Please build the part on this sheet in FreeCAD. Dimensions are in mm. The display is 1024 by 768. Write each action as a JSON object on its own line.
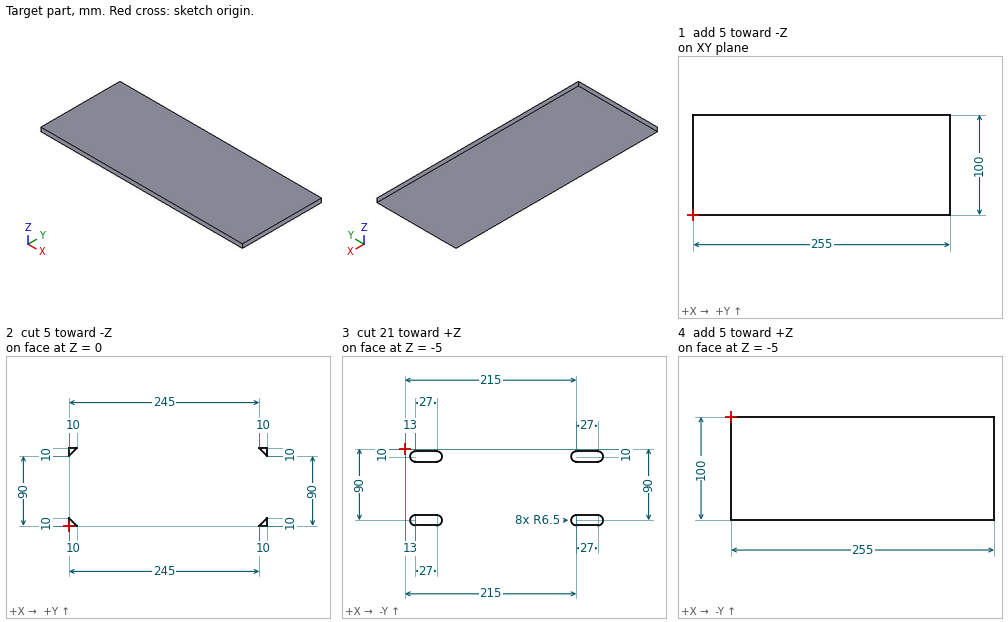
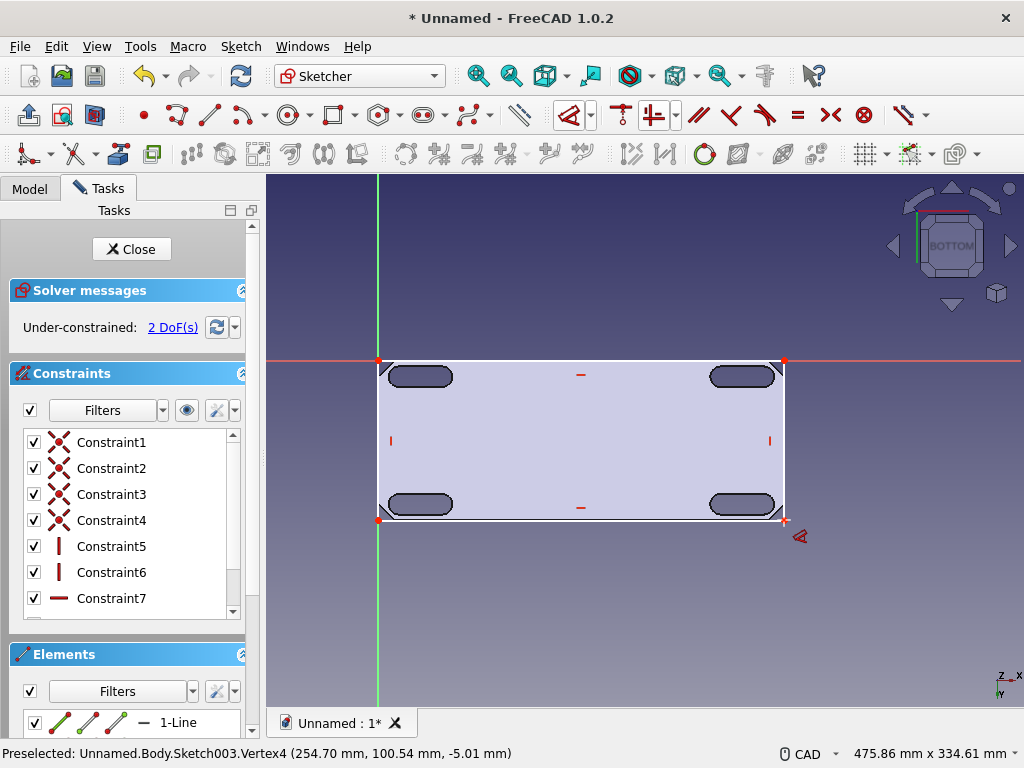
{"action": "left_click", "coordinate": [378, 409]}
{"action": "left_click", "coordinate": [344, 441]}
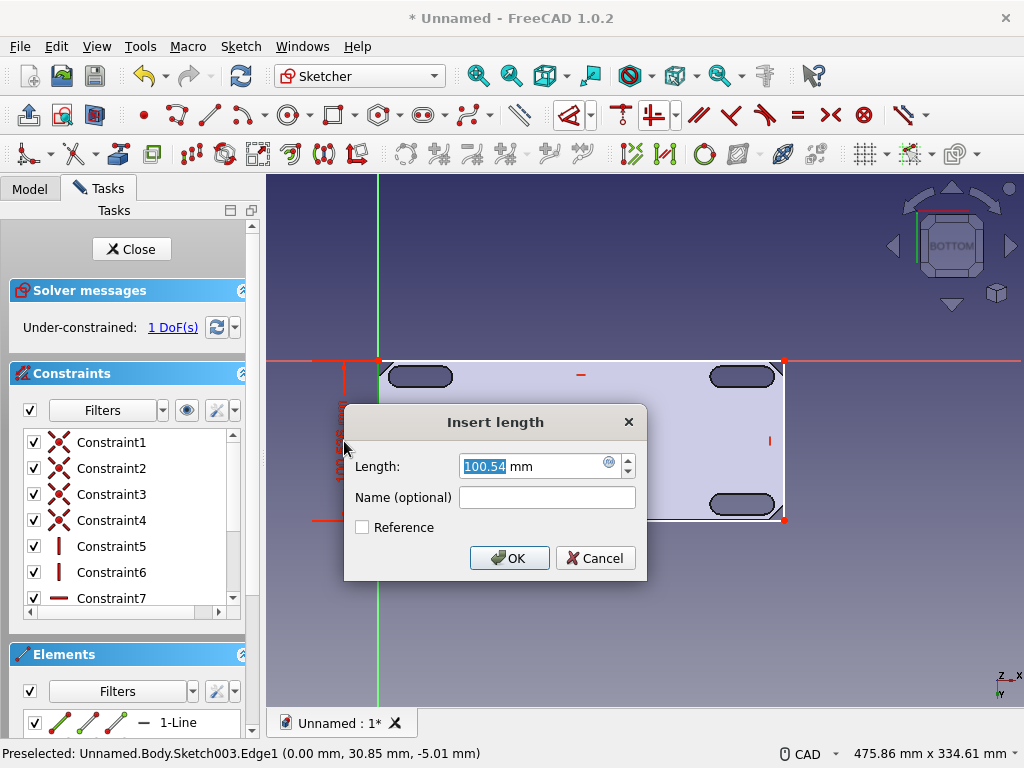
{"action": "type", "text": "100"}
{"action": "key", "text": "Return"}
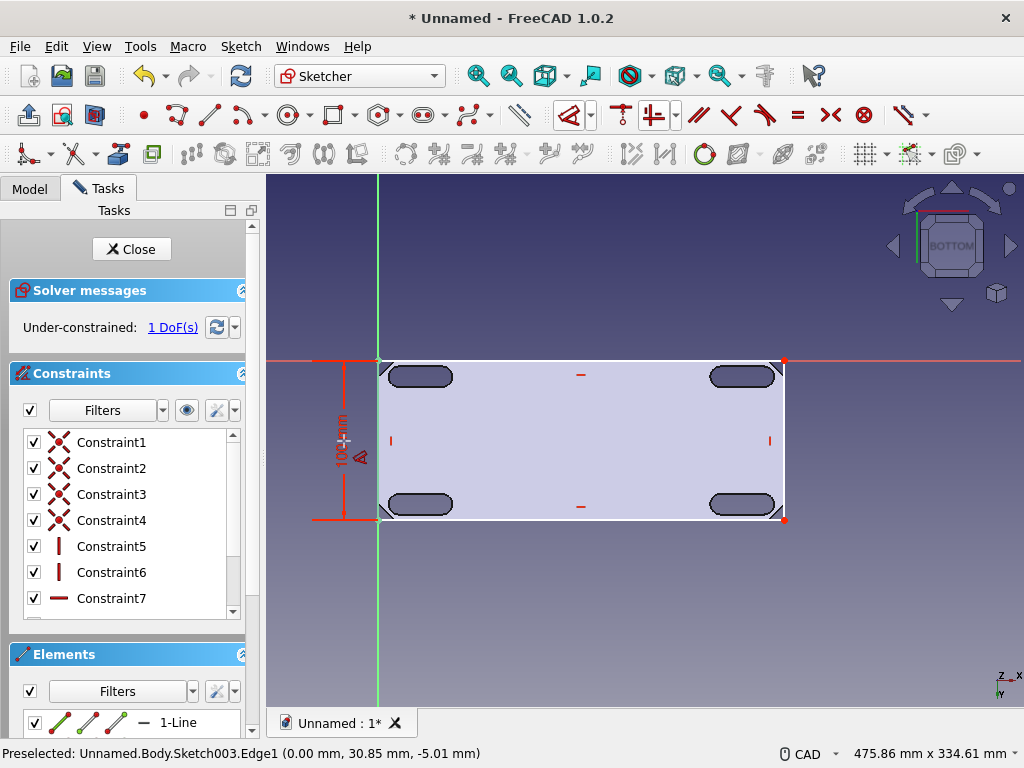
{"action": "left_click", "coordinate": [500, 520]}
{"action": "left_click", "coordinate": [581, 554]}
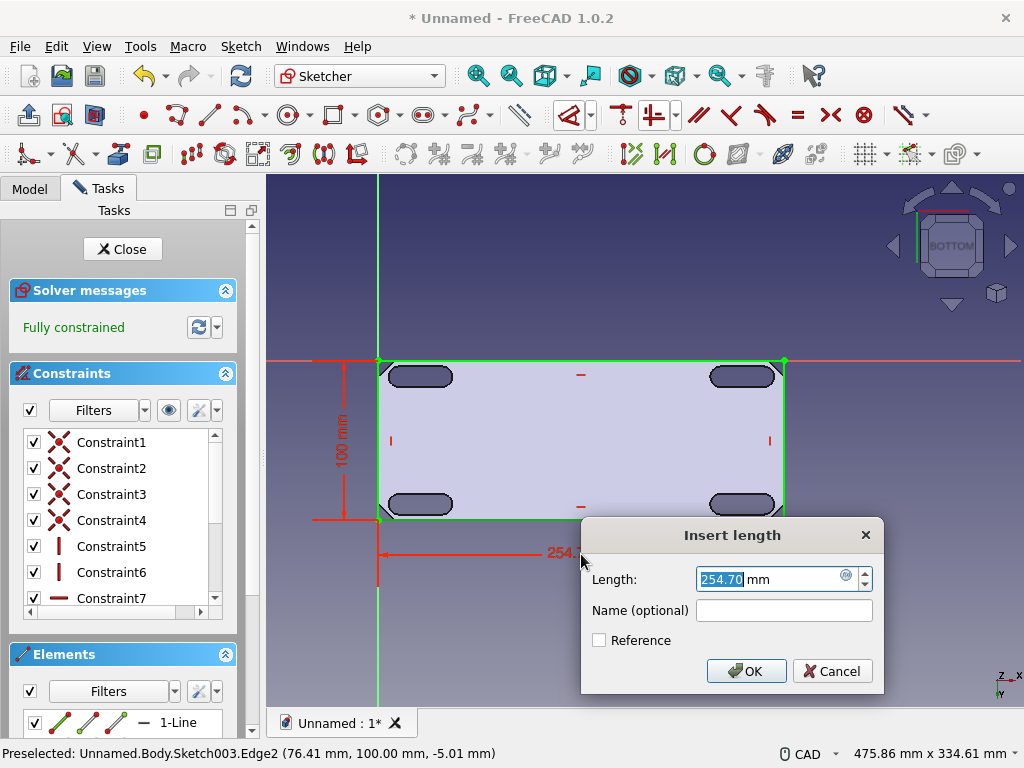
{"action": "type", "text": "255"}
{"action": "key", "text": "Return"}
{"action": "key", "text": "Escape"}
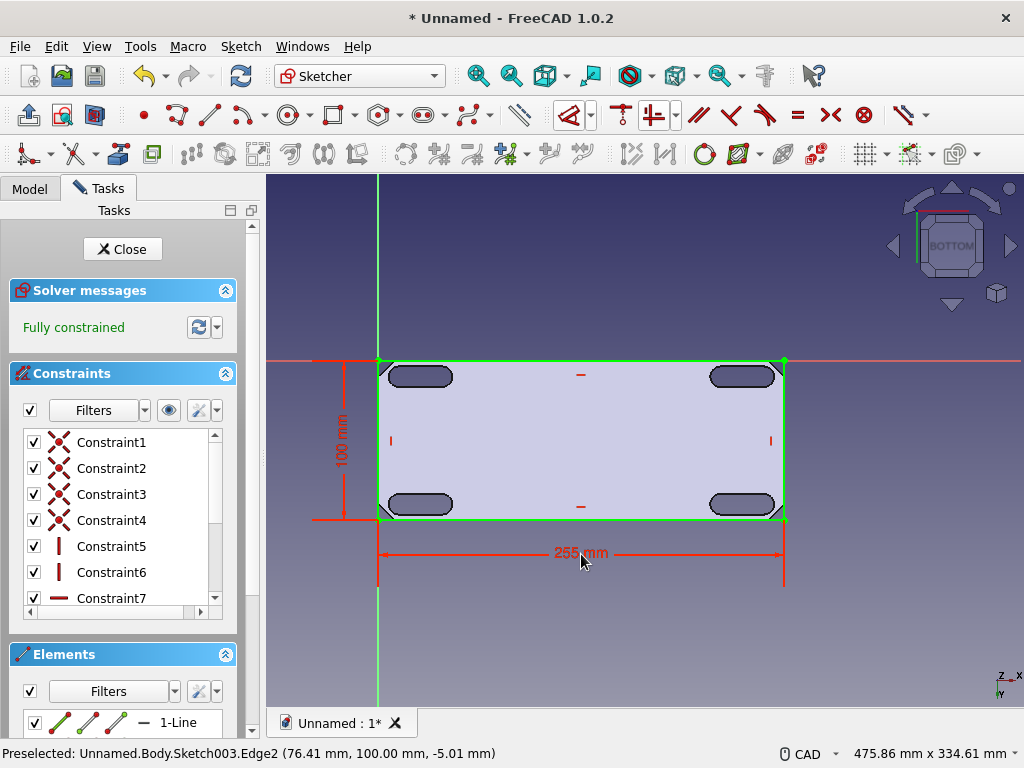
{"action": "left_click", "coordinate": [123, 249]}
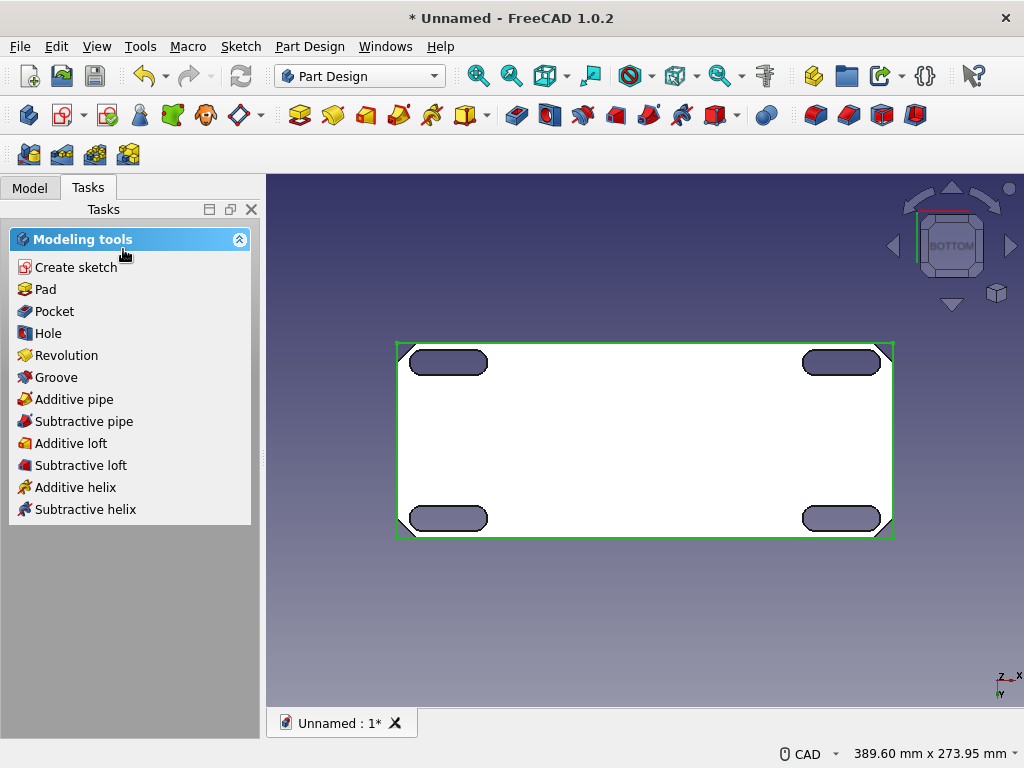
{"action": "left_click", "coordinate": [300, 116]}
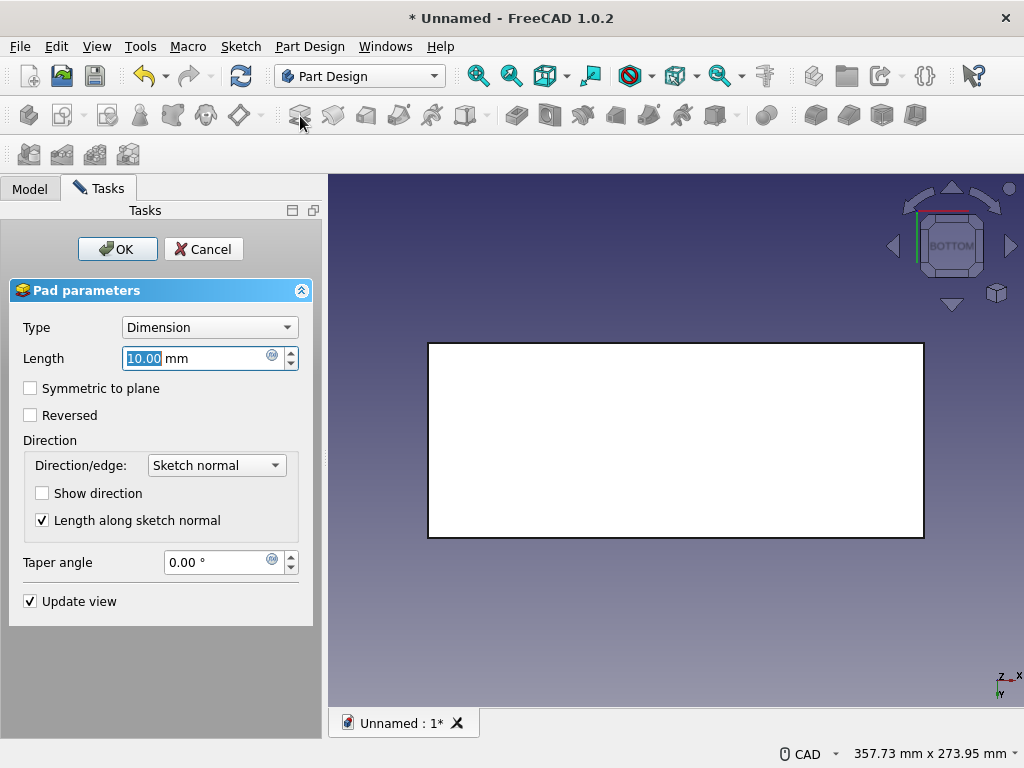
{"action": "type", "text": "5"}
{"action": "key", "text": "Tab"}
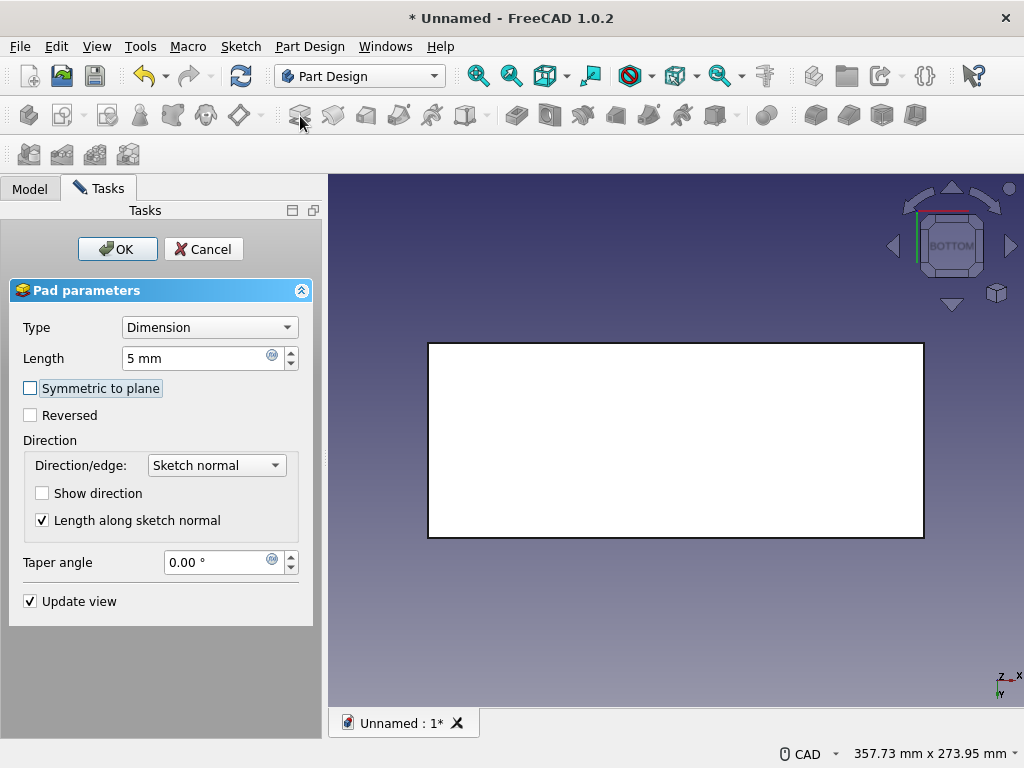
{"action": "left_click", "coordinate": [31, 415]}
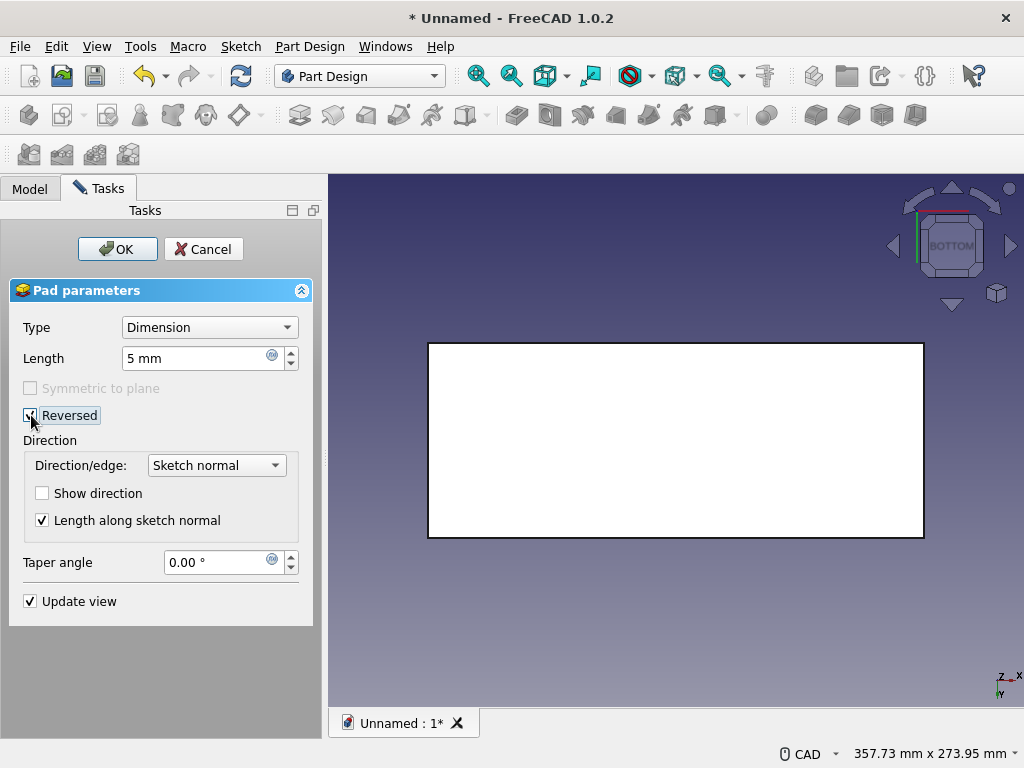
{"action": "left_click", "coordinate": [118, 249]}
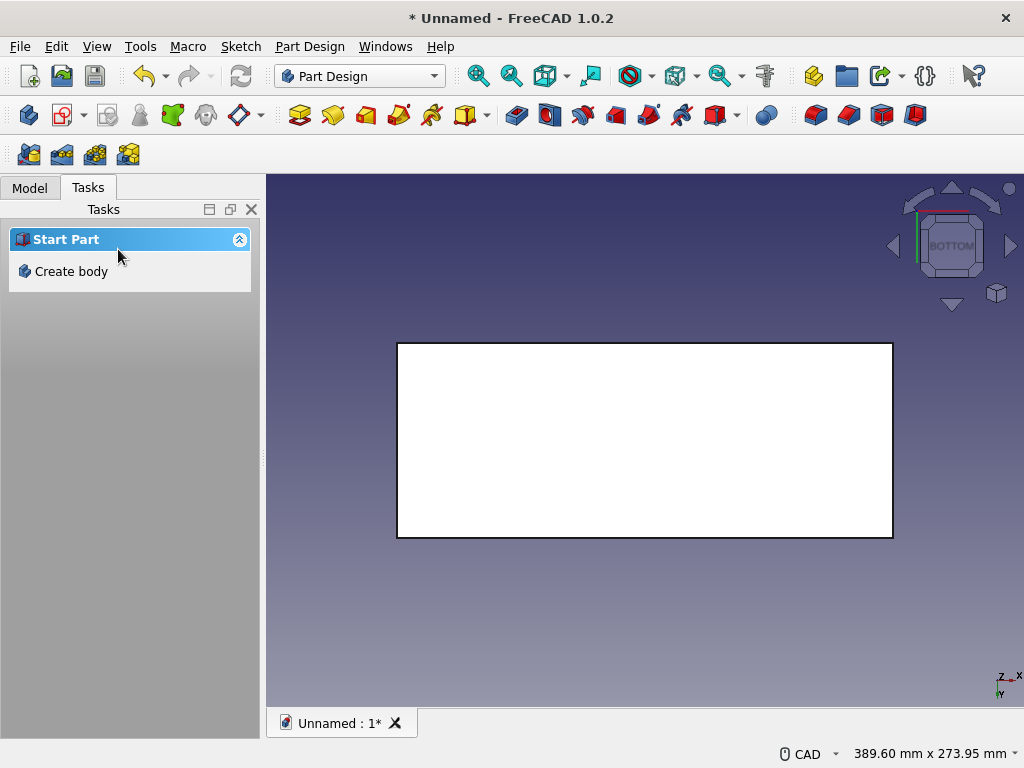
{"action": "key", "text": "0"}